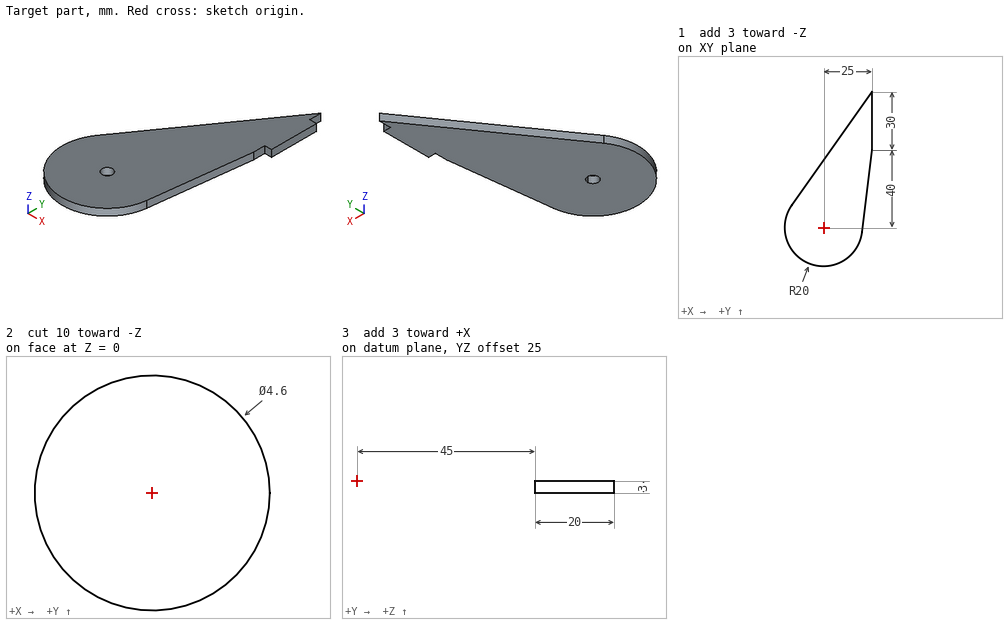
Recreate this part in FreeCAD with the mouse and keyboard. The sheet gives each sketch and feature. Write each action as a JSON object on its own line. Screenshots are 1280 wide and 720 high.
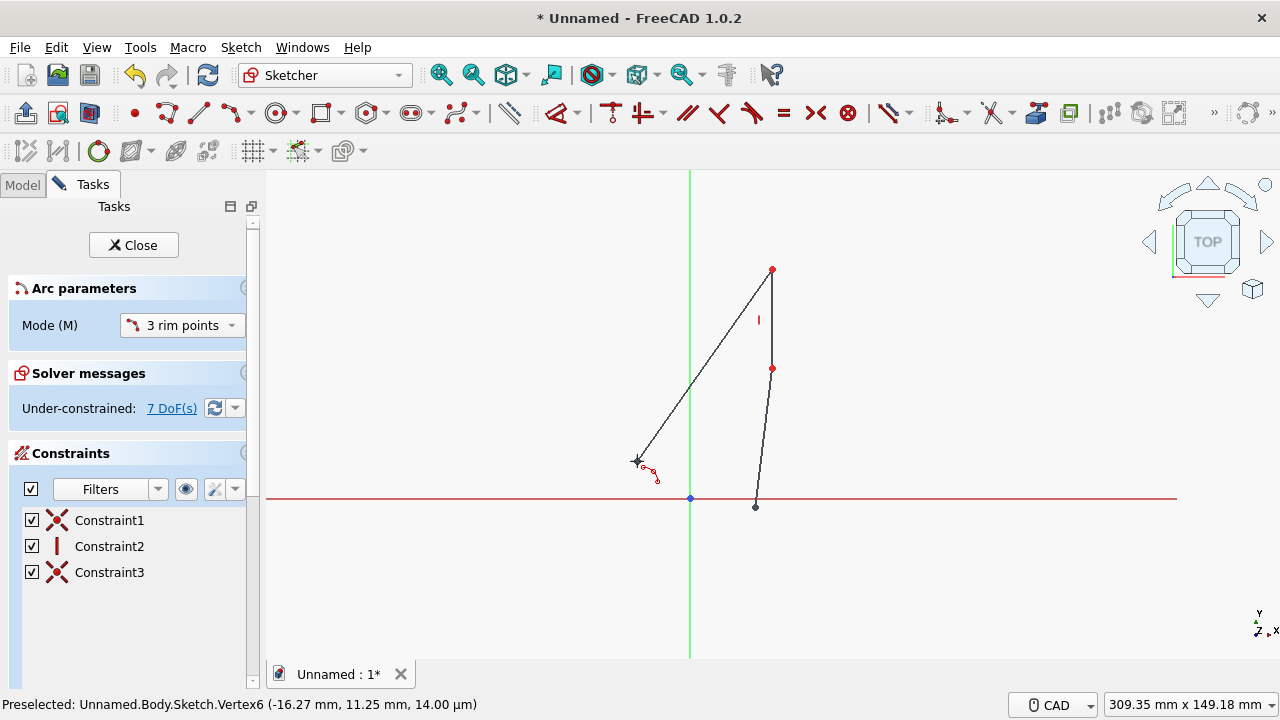
{"action": "left_click", "coordinate": [637, 462]}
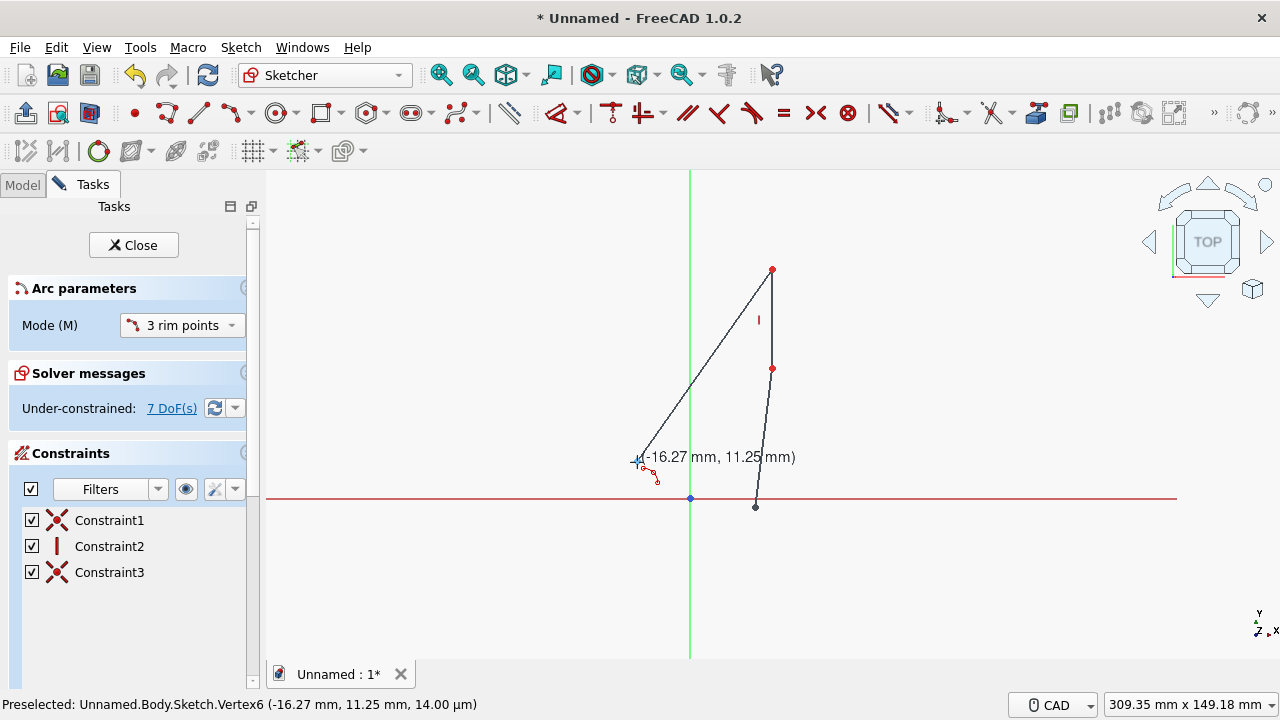
{"action": "scroll", "coordinate": [755, 507], "scroll_direction": "up", "scroll_amount": 4}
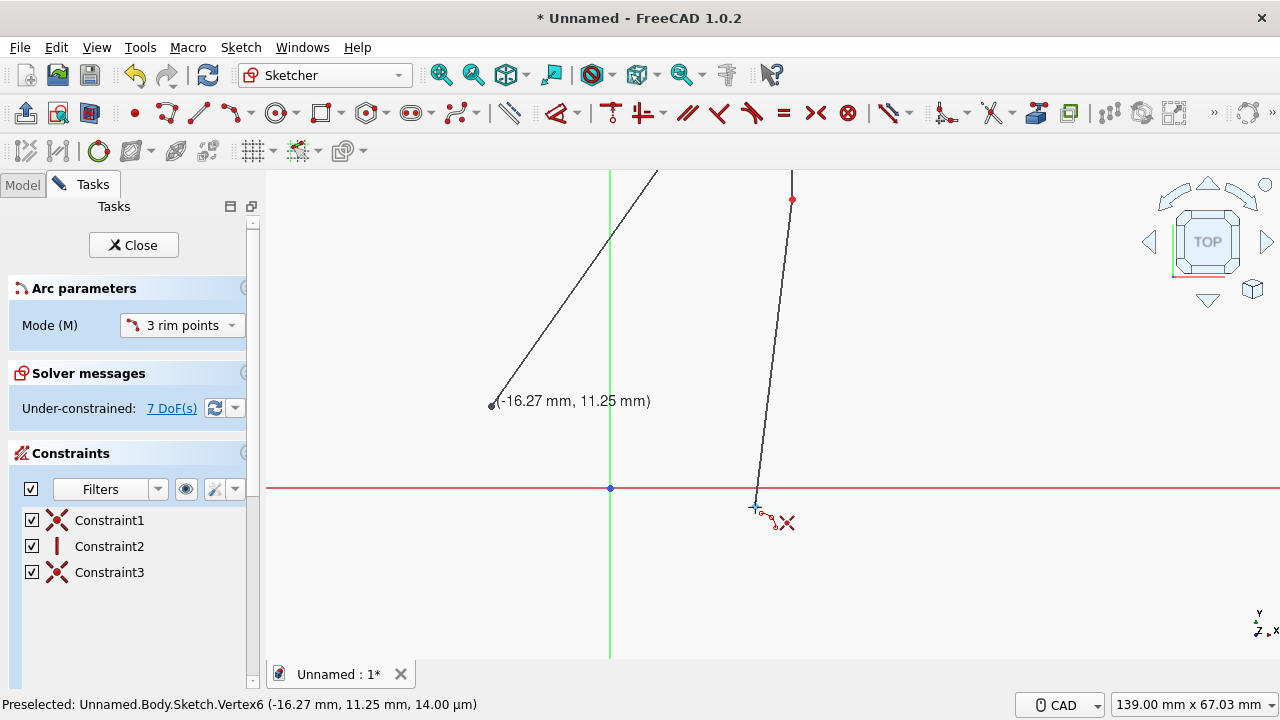
{"action": "left_click", "coordinate": [755, 506]}
{"action": "left_click", "coordinate": [558, 624]}
{"action": "key", "text": "Escape"}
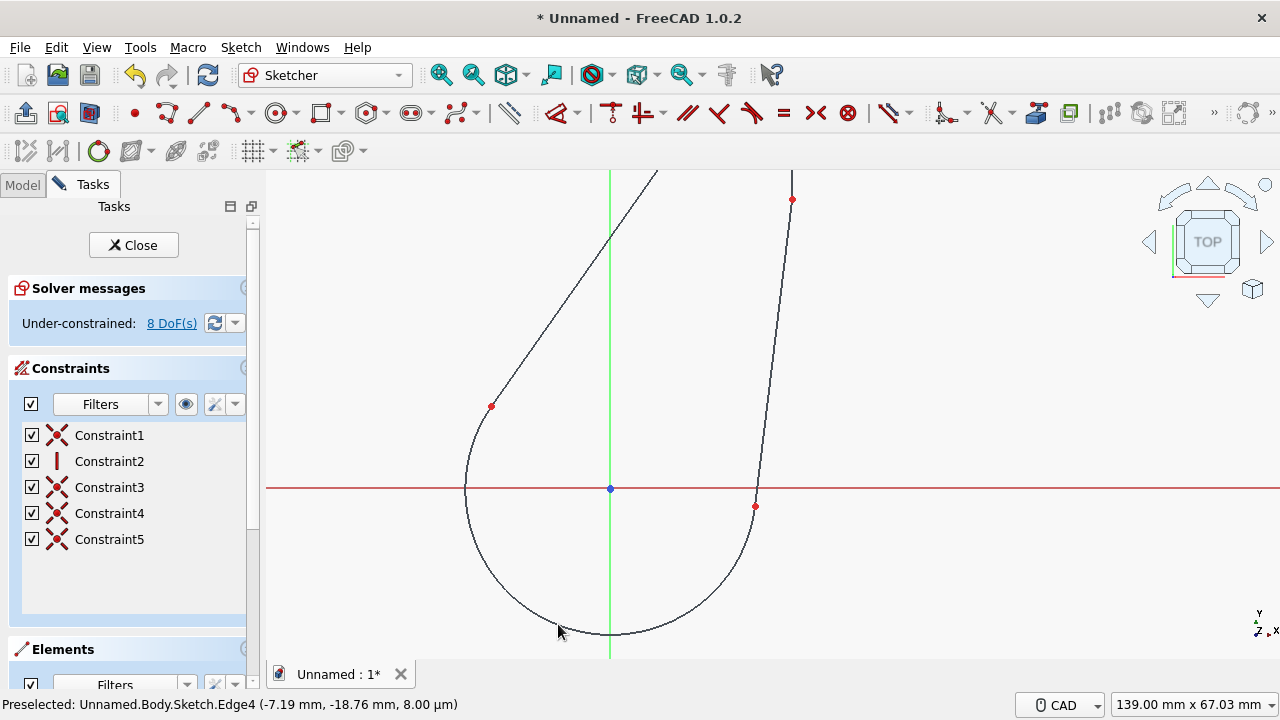
{"action": "left_click", "coordinate": [766, 414]}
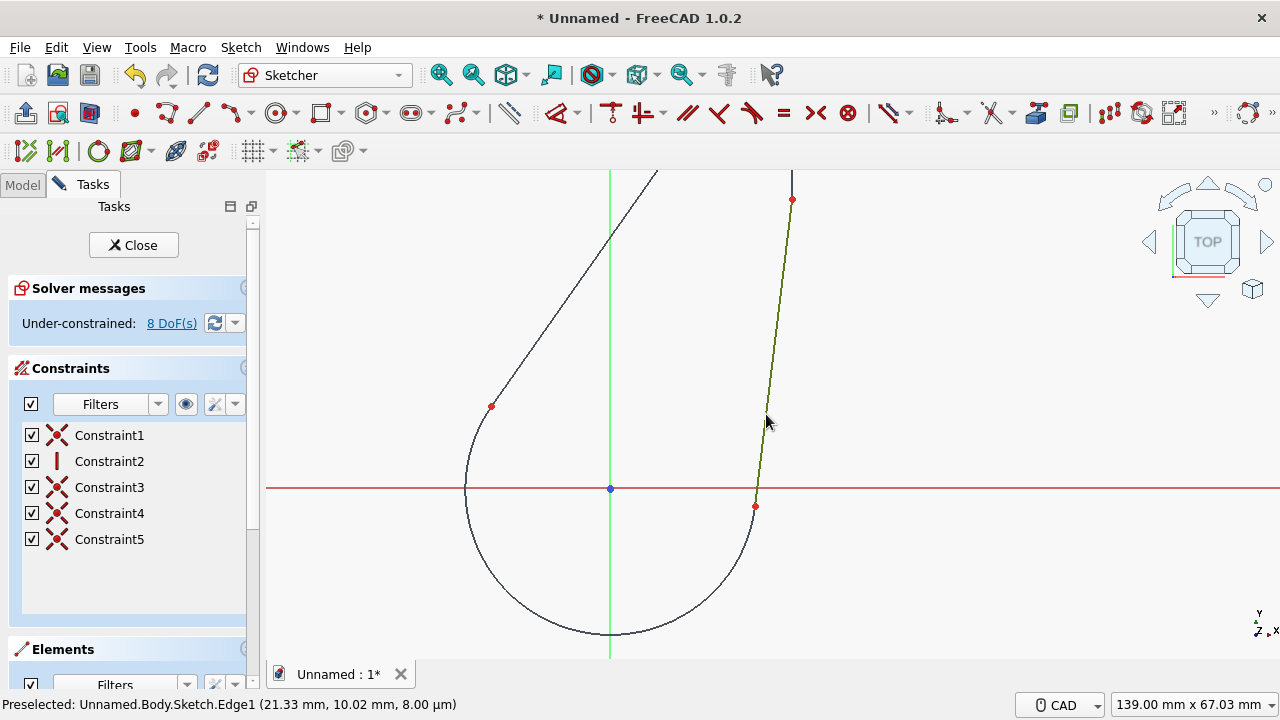
{"action": "left_click", "coordinate": [482, 557]}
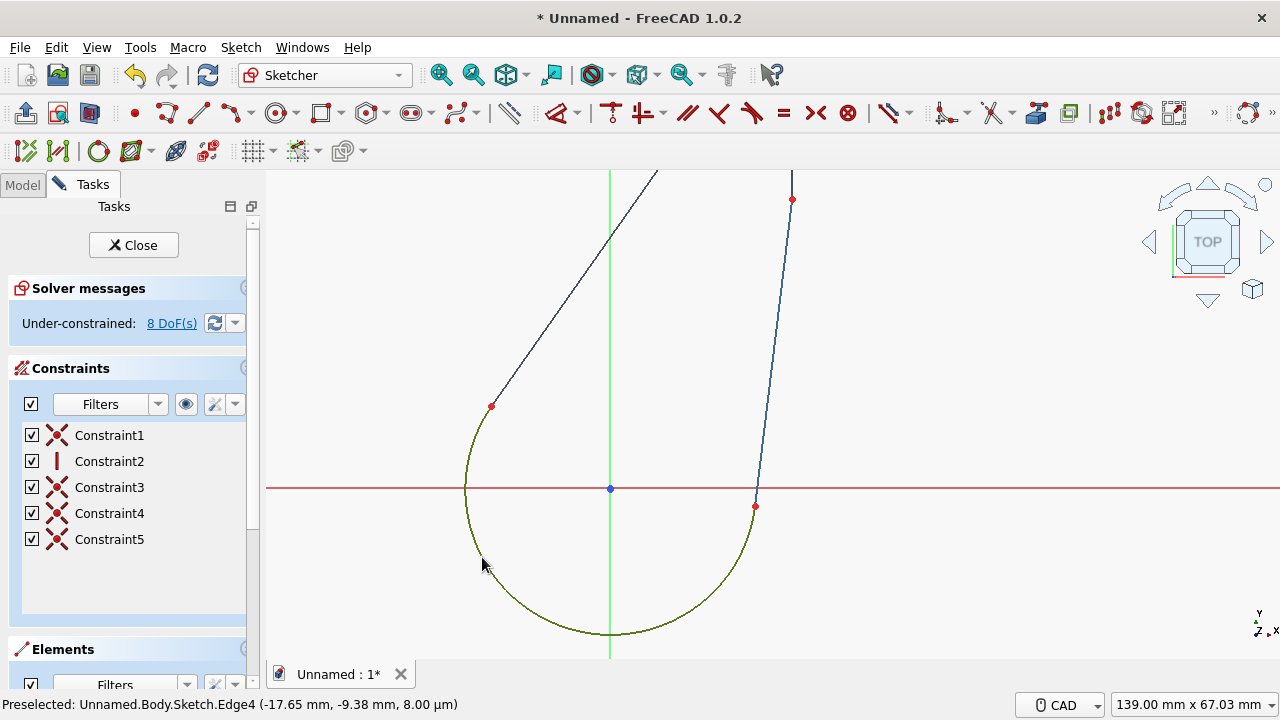
{"action": "left_click", "coordinate": [752, 114]}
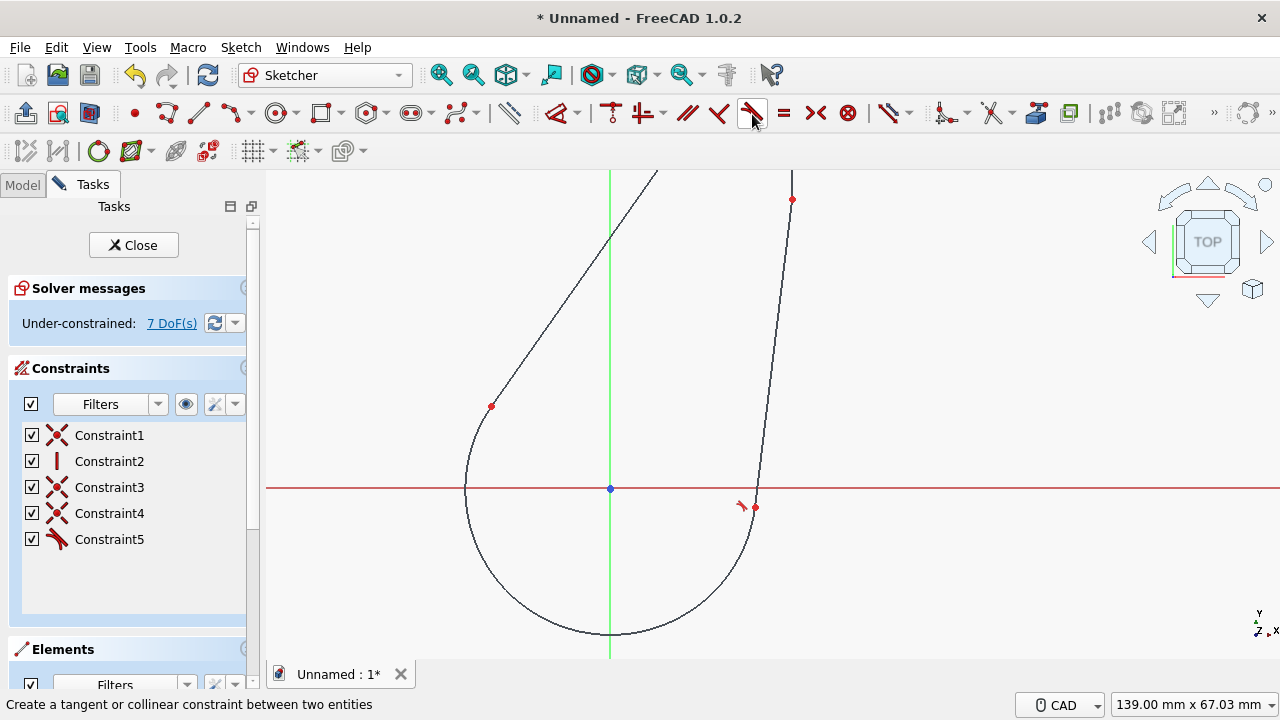
{"action": "left_click", "coordinate": [582, 278]}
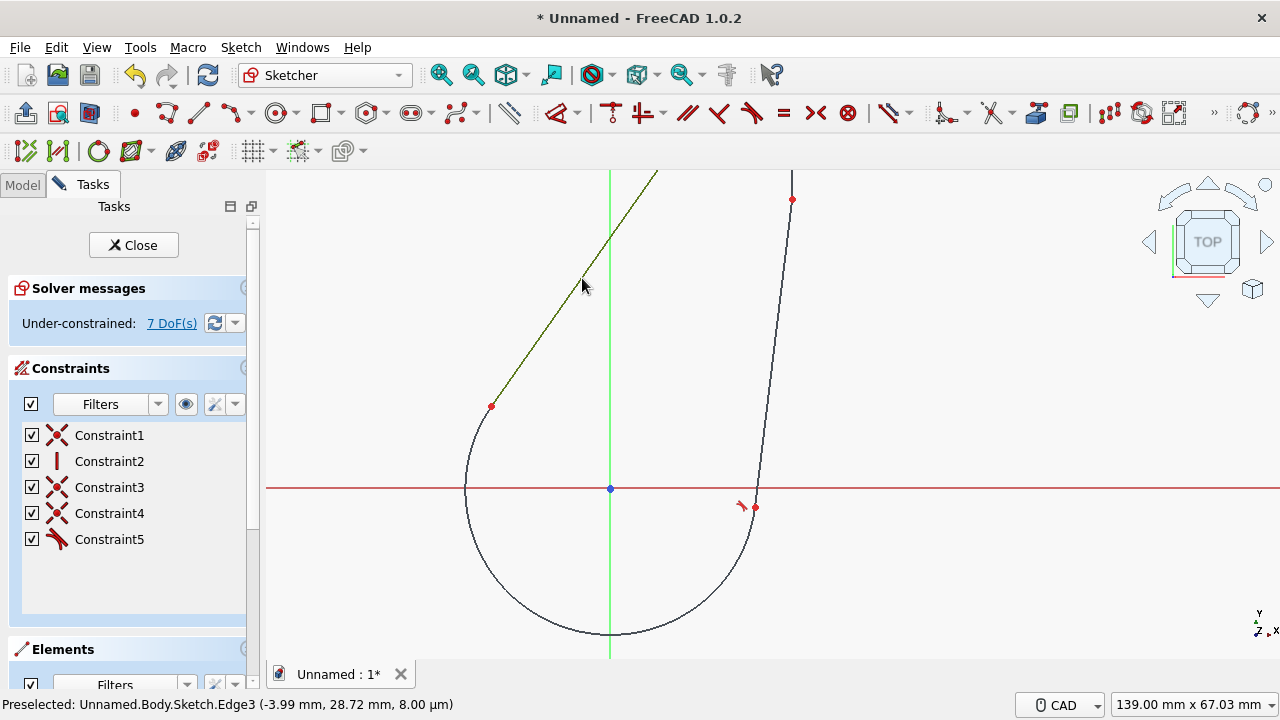
{"action": "left_click", "coordinate": [482, 556]}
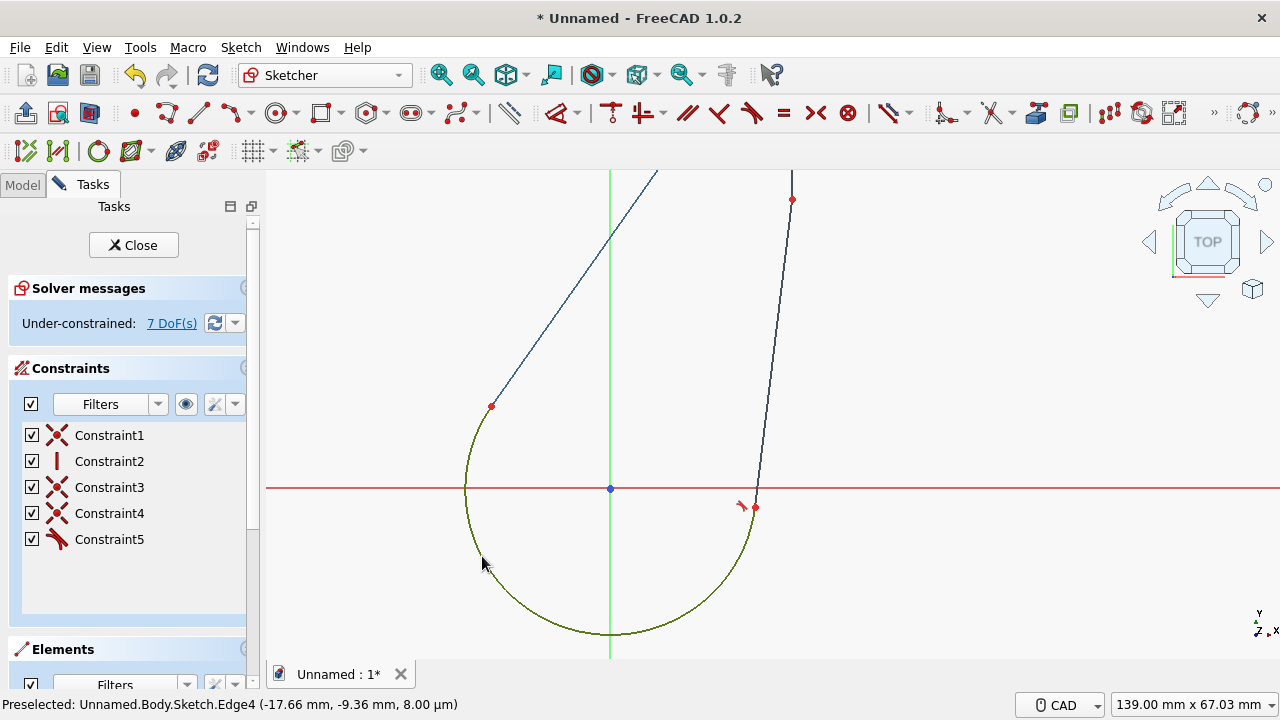
{"action": "key", "text": "t"}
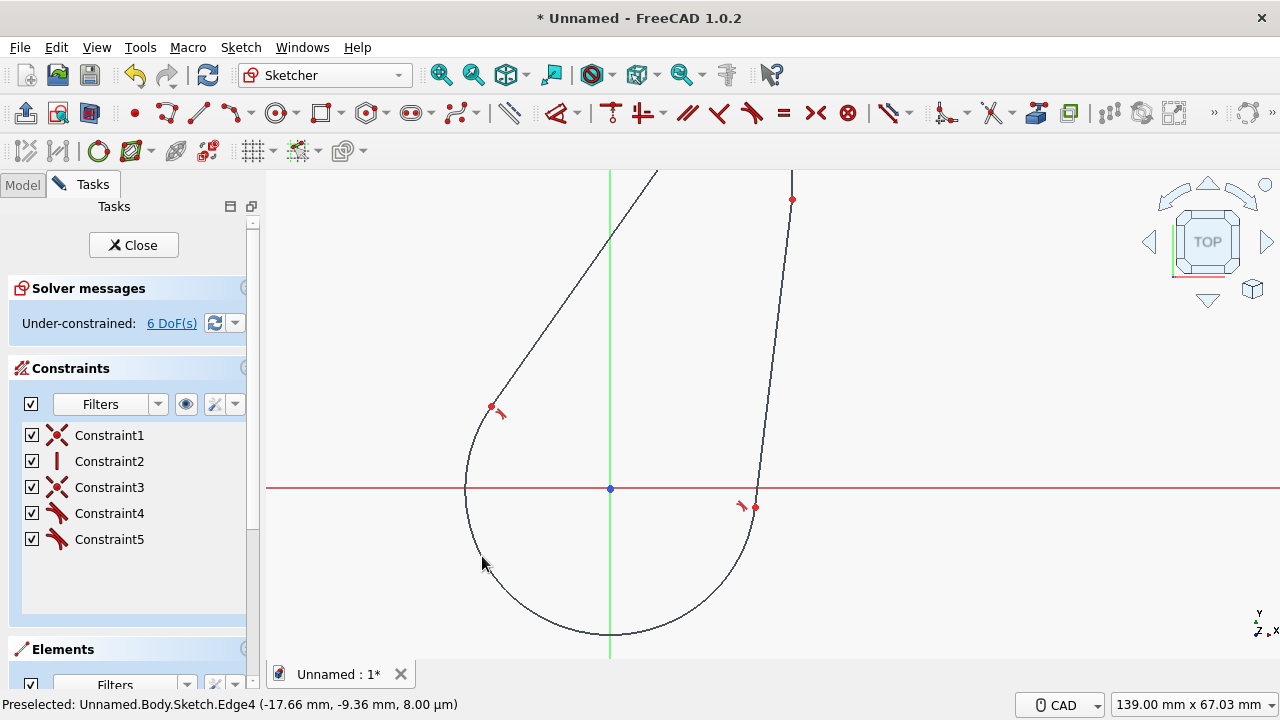
{"action": "left_click_drag", "start_coordinate": [600, 478], "coordinate": [621, 500]}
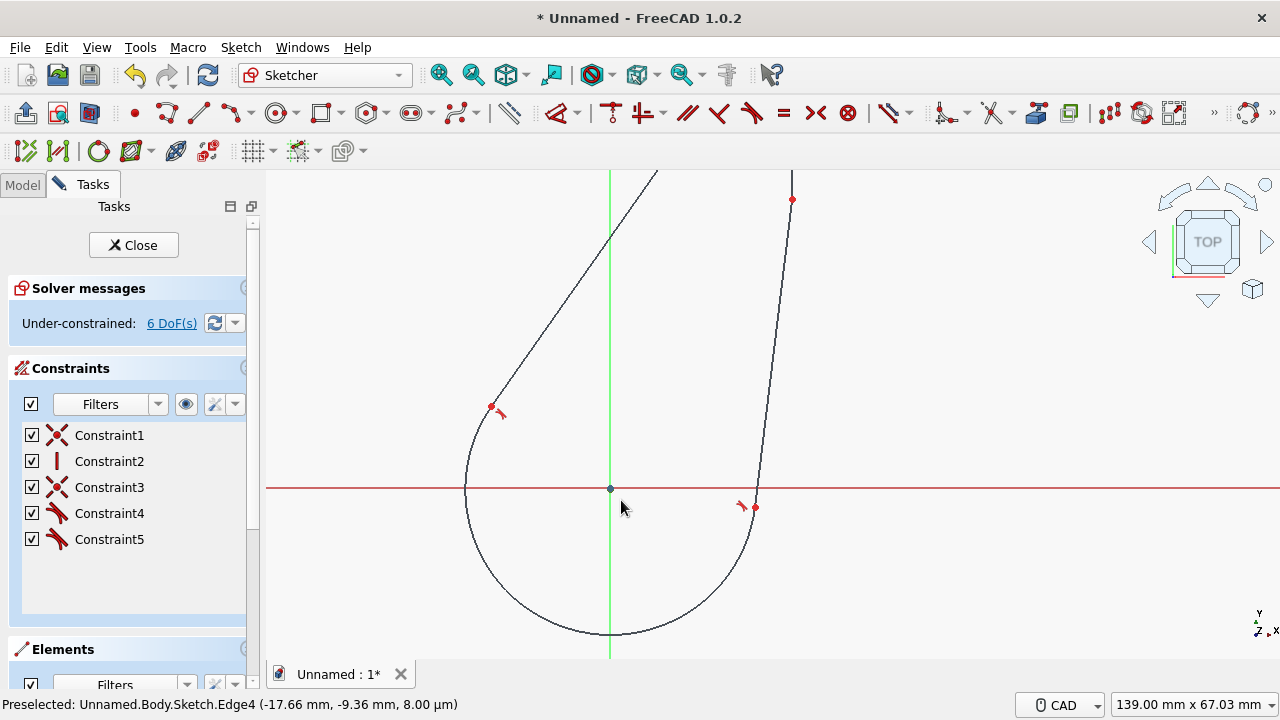
{"action": "key", "text": "c"}